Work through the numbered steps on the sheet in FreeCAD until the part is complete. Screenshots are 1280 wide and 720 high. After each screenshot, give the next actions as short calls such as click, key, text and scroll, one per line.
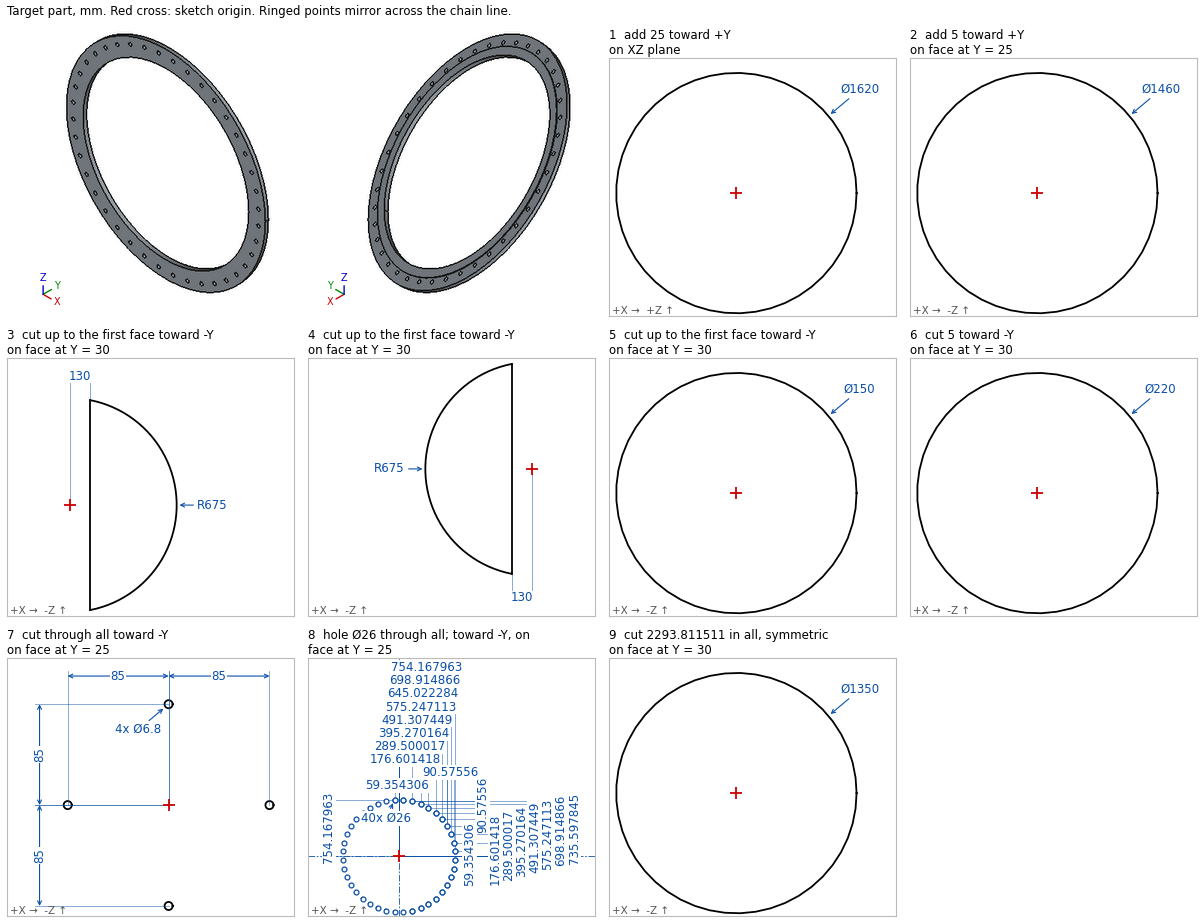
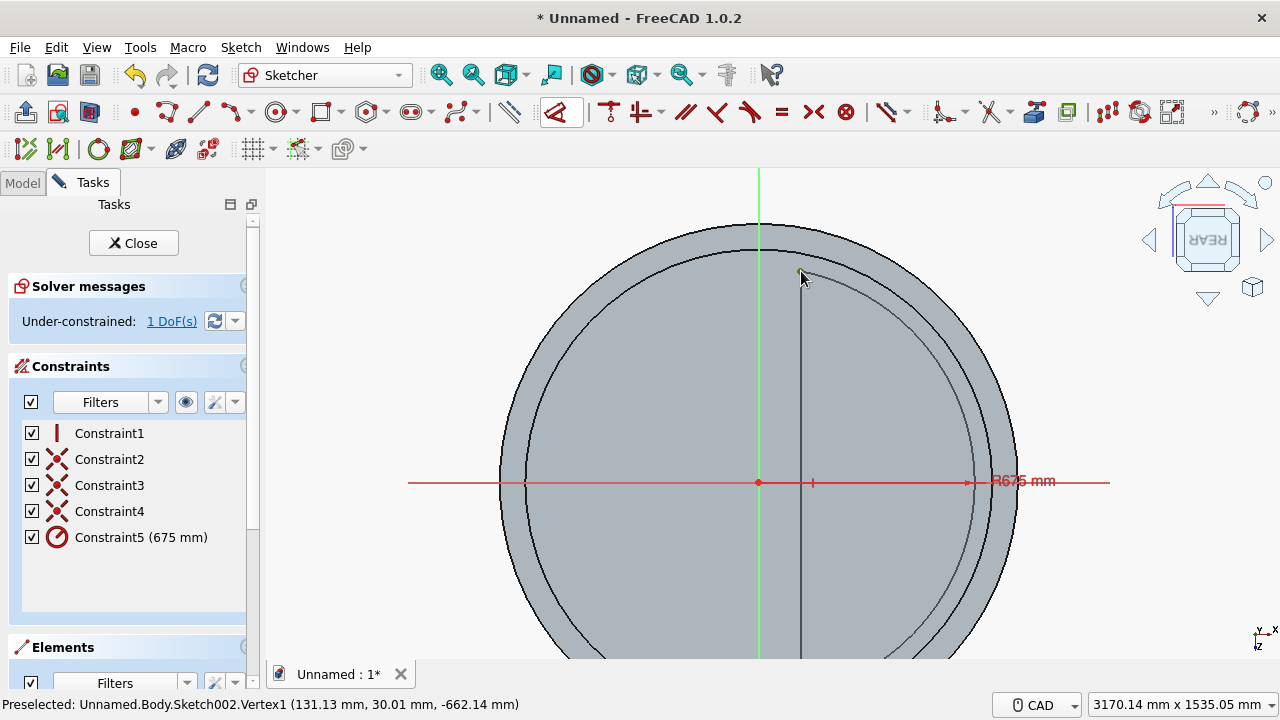
key(l)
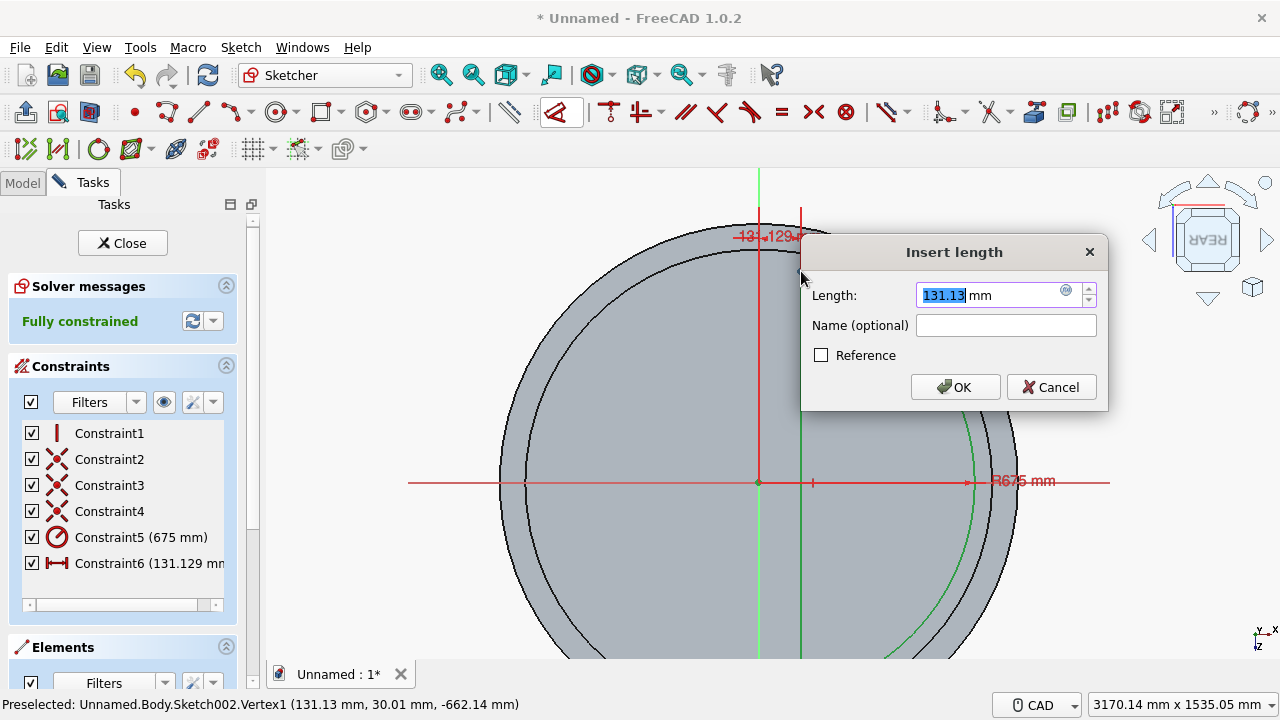
text(130)
key(Return)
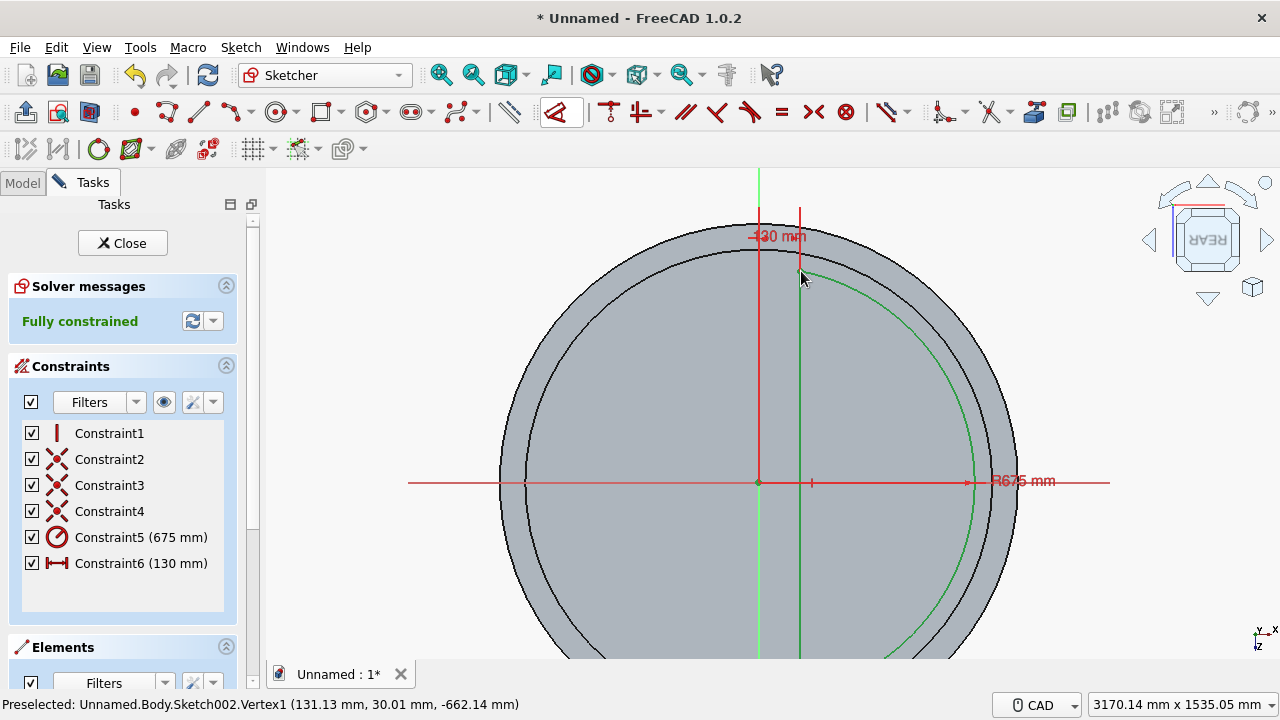
click(123, 243)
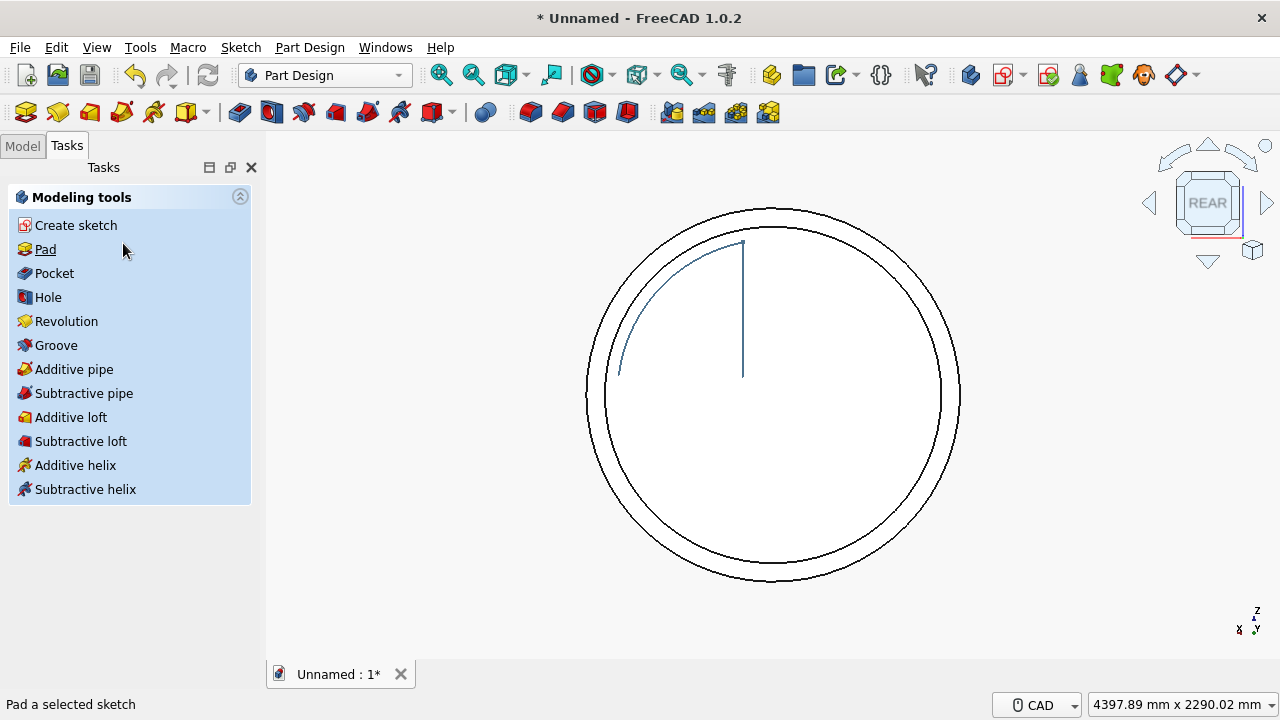
click(240, 112)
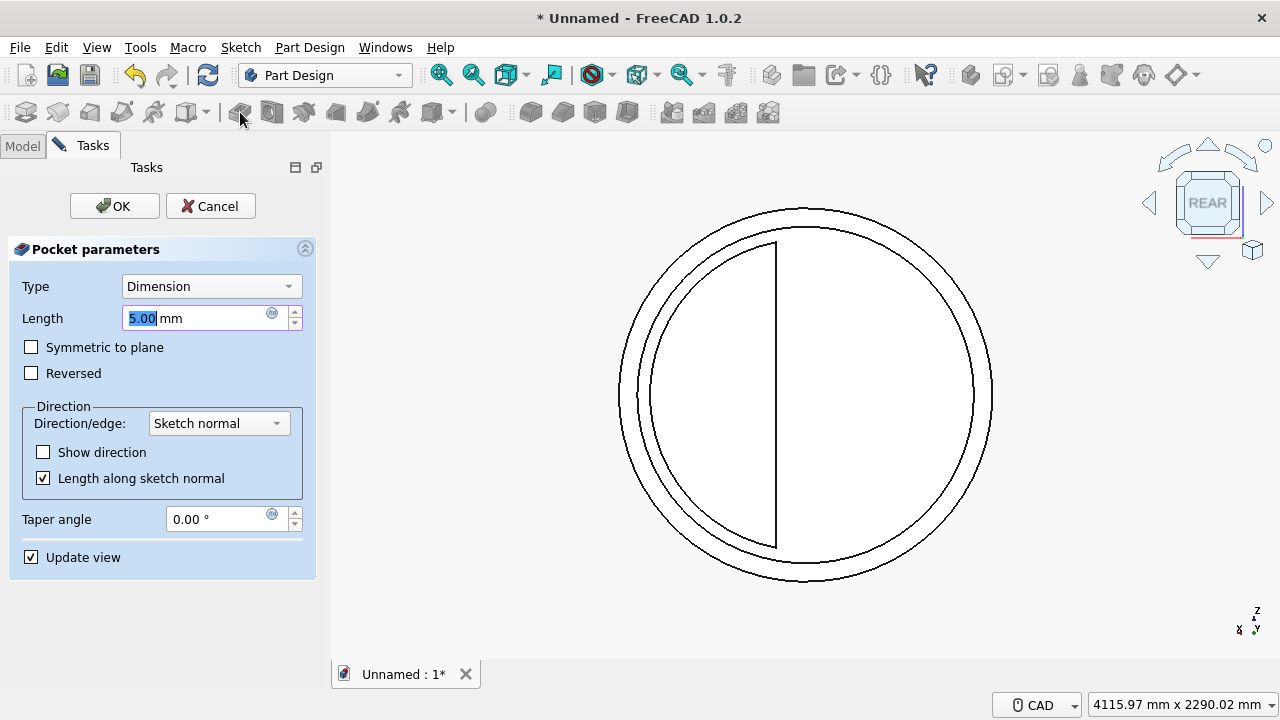
click(212, 286)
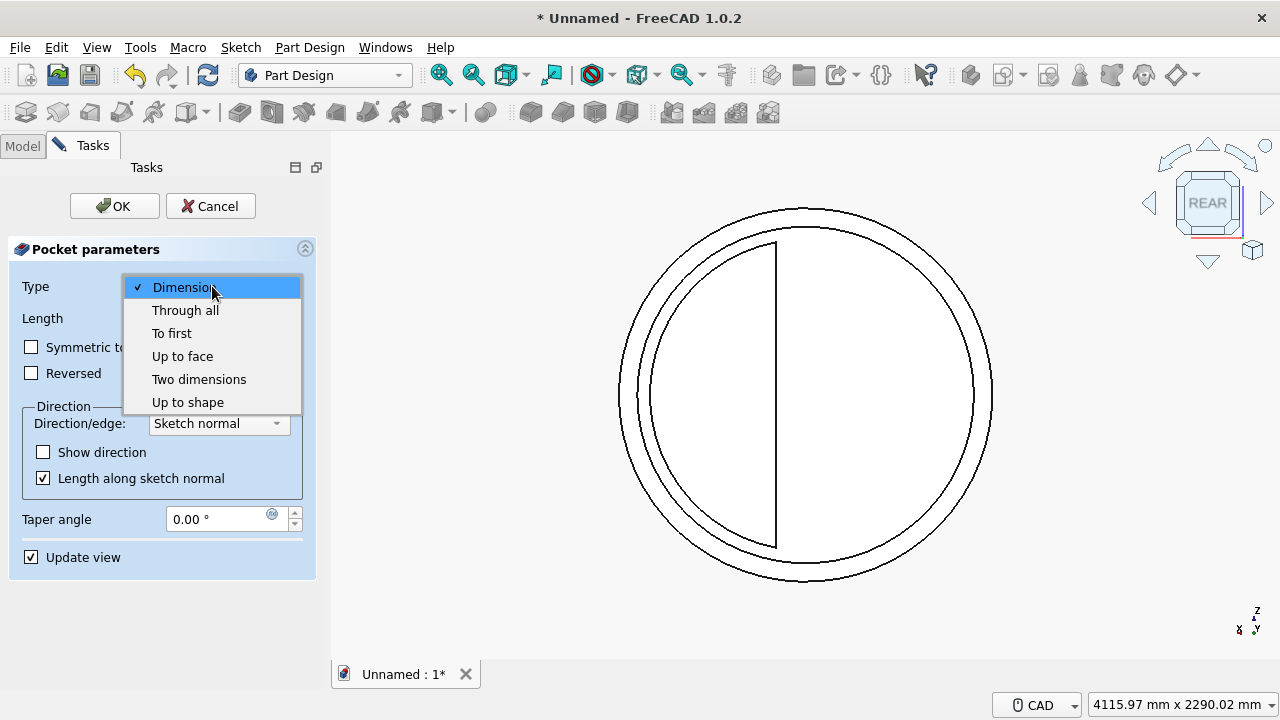
click(212, 334)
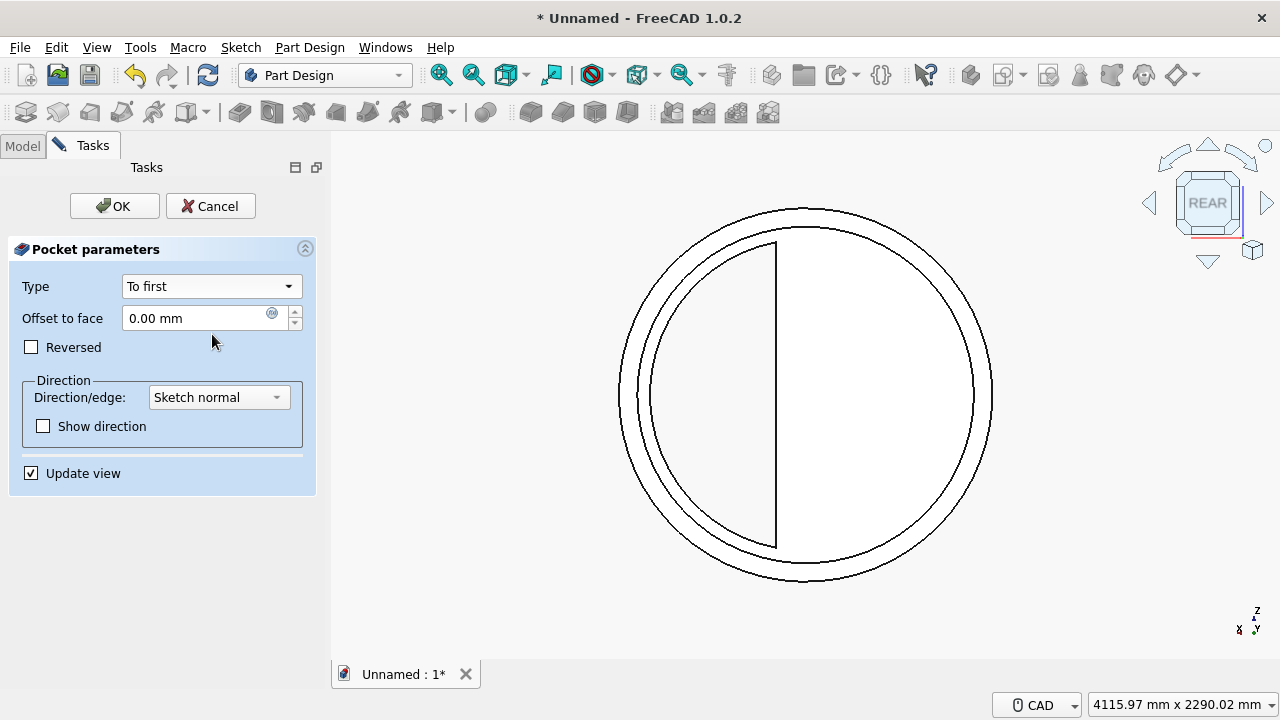
click(115, 206)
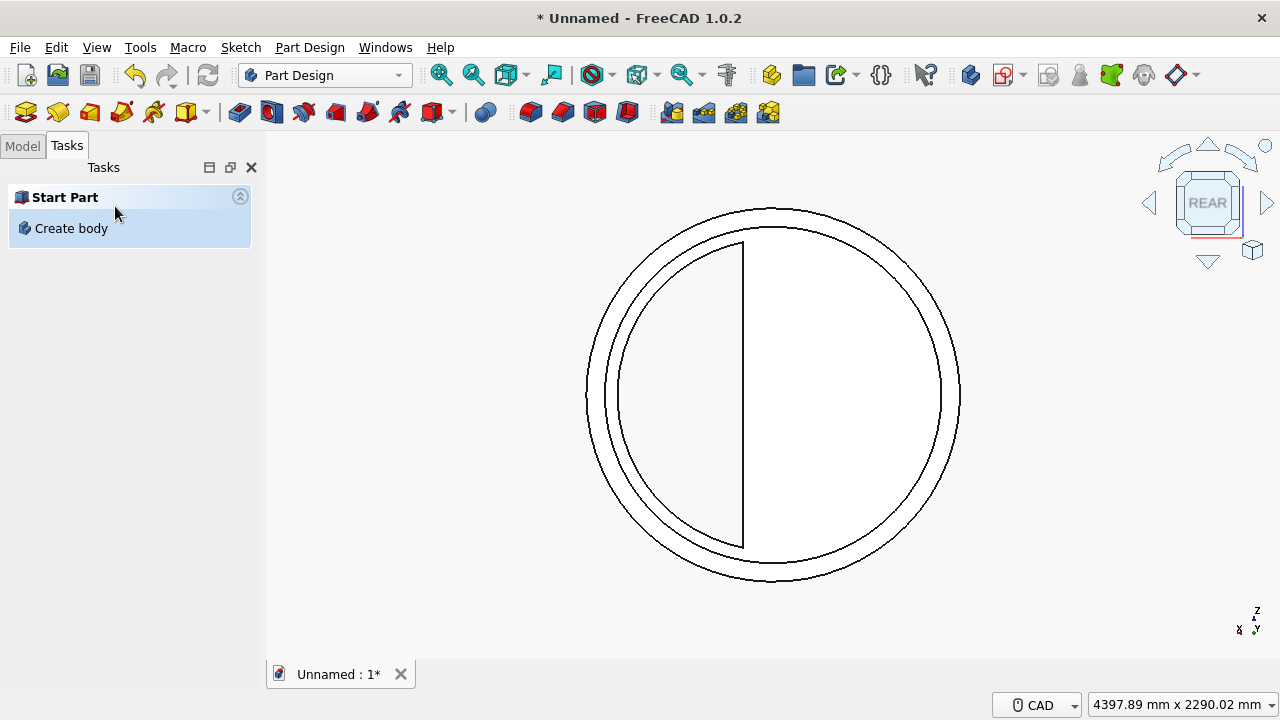
click(821, 442)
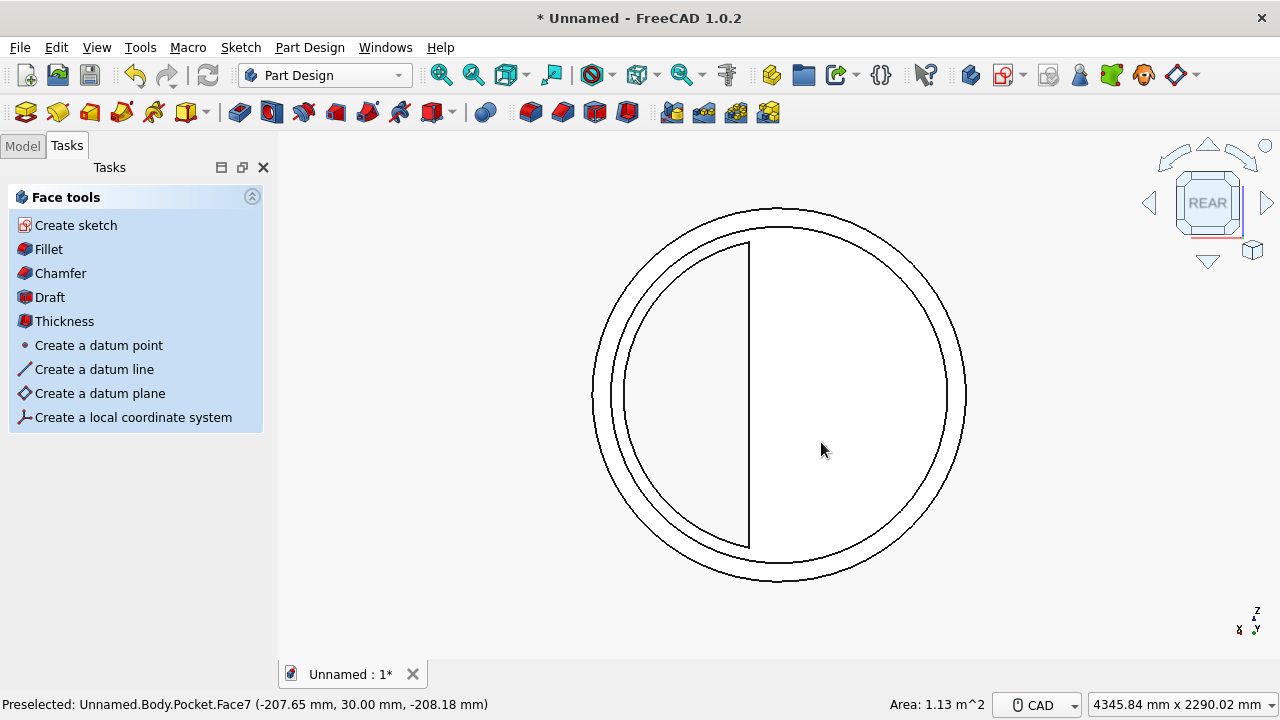
click(1004, 76)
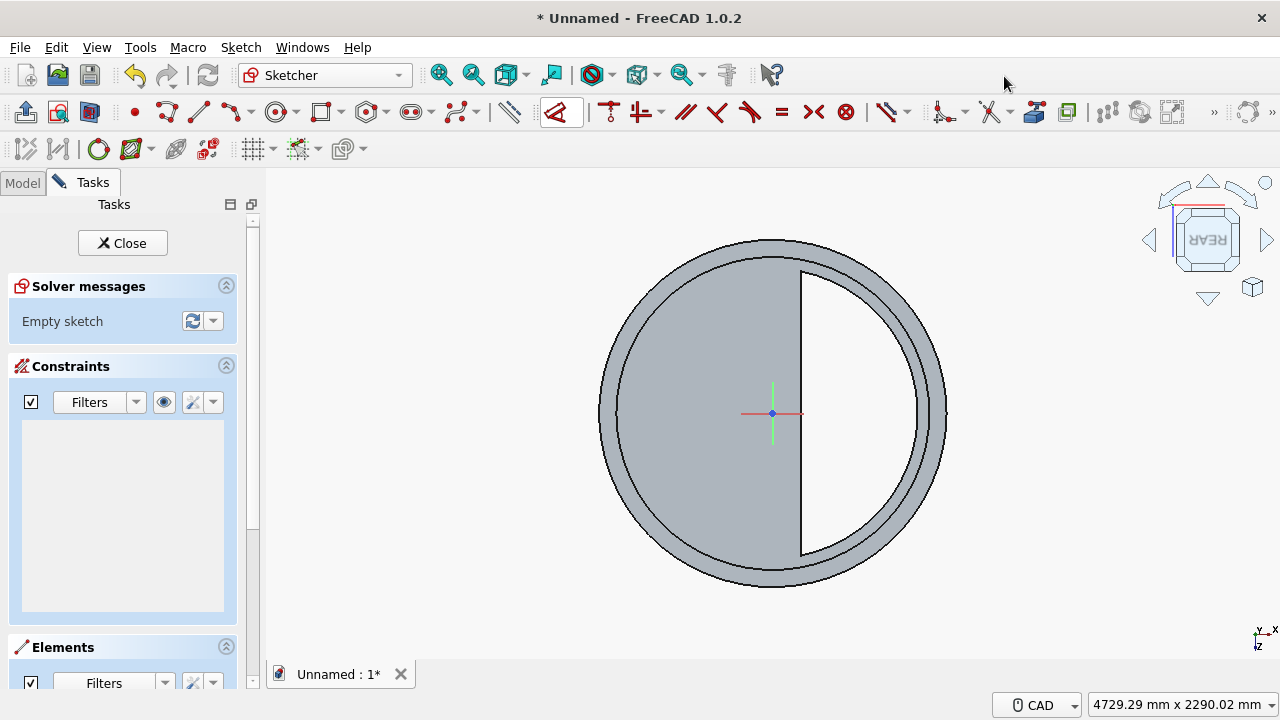
click(200, 112)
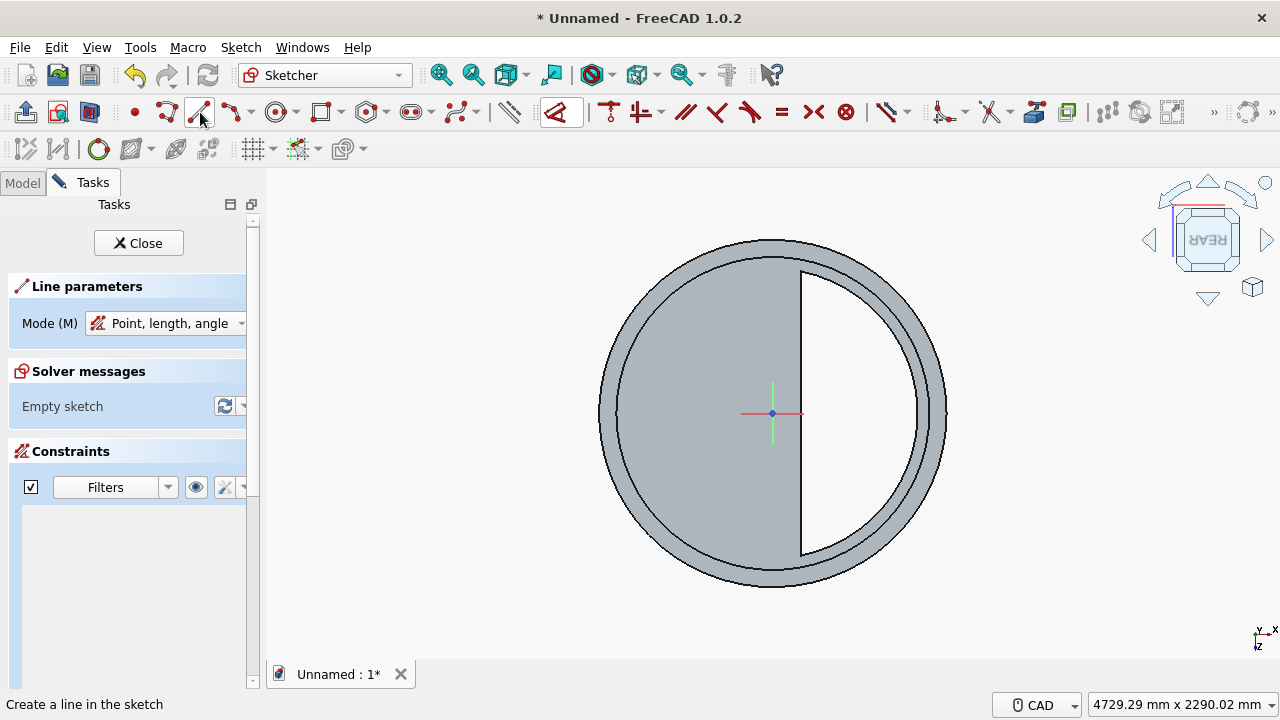
click(745, 556)
click(745, 271)